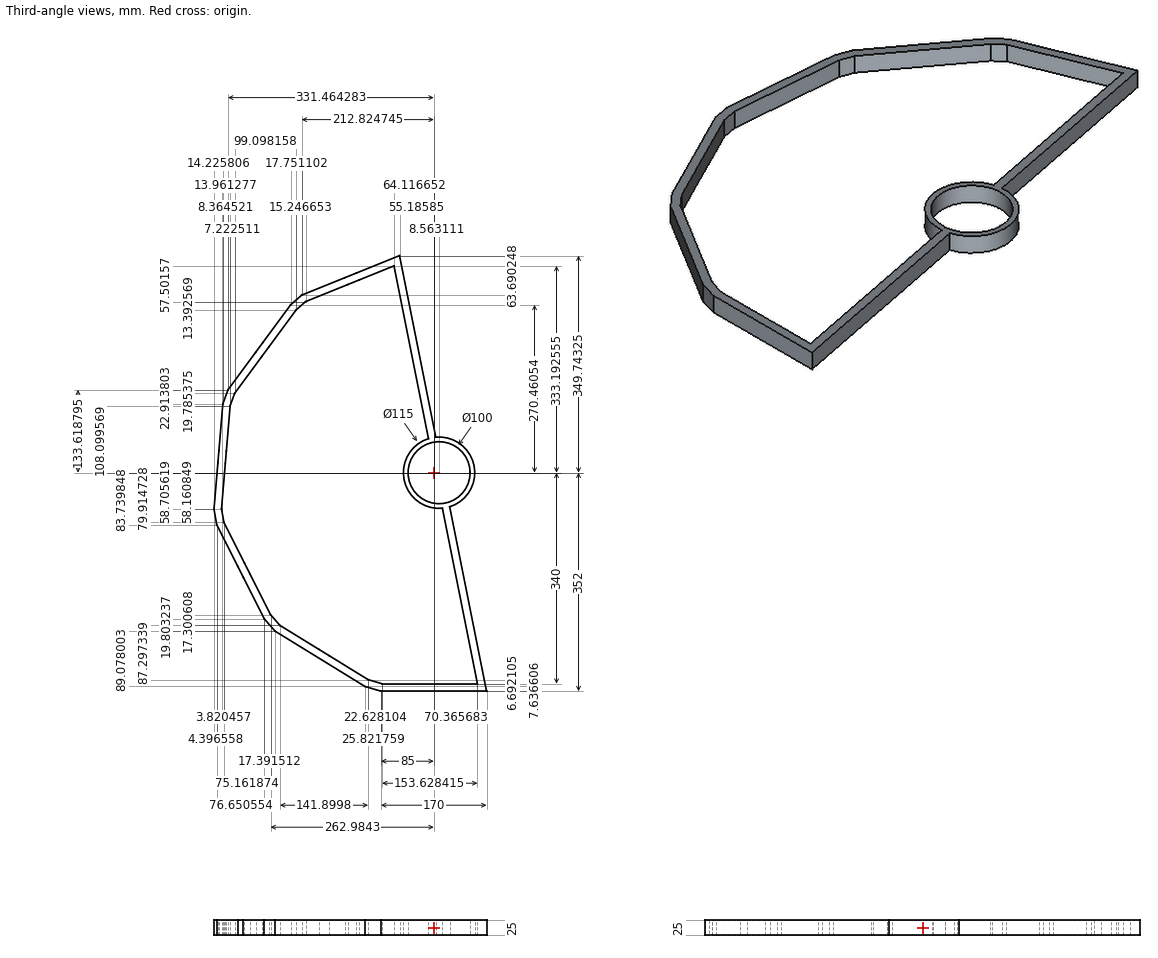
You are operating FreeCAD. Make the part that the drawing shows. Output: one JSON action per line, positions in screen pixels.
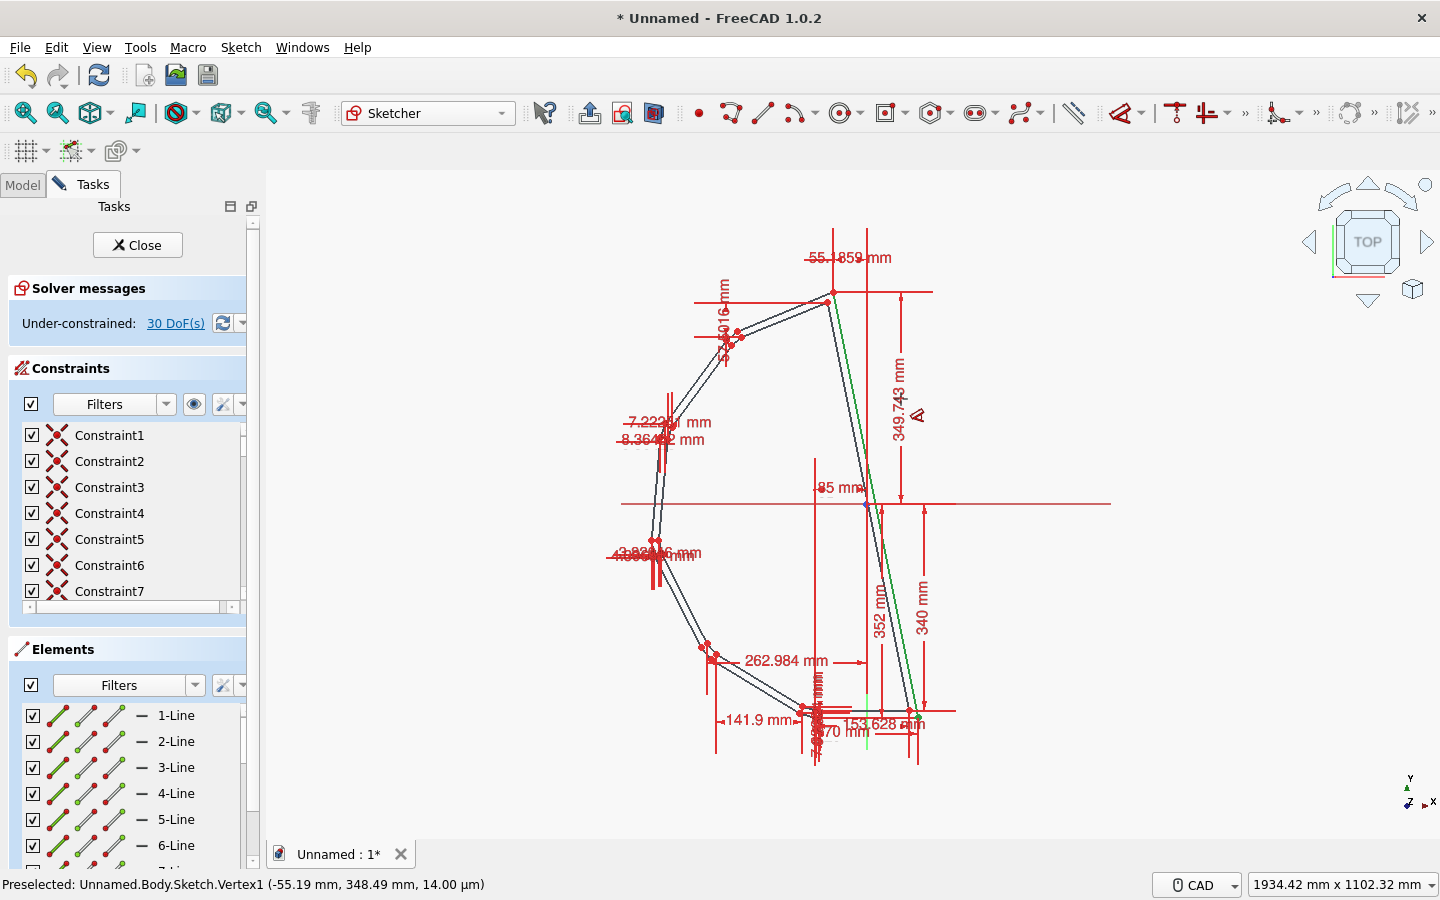
{"action": "scroll", "coordinate": [726, 341], "scroll_direction": "up", "scroll_amount": 3}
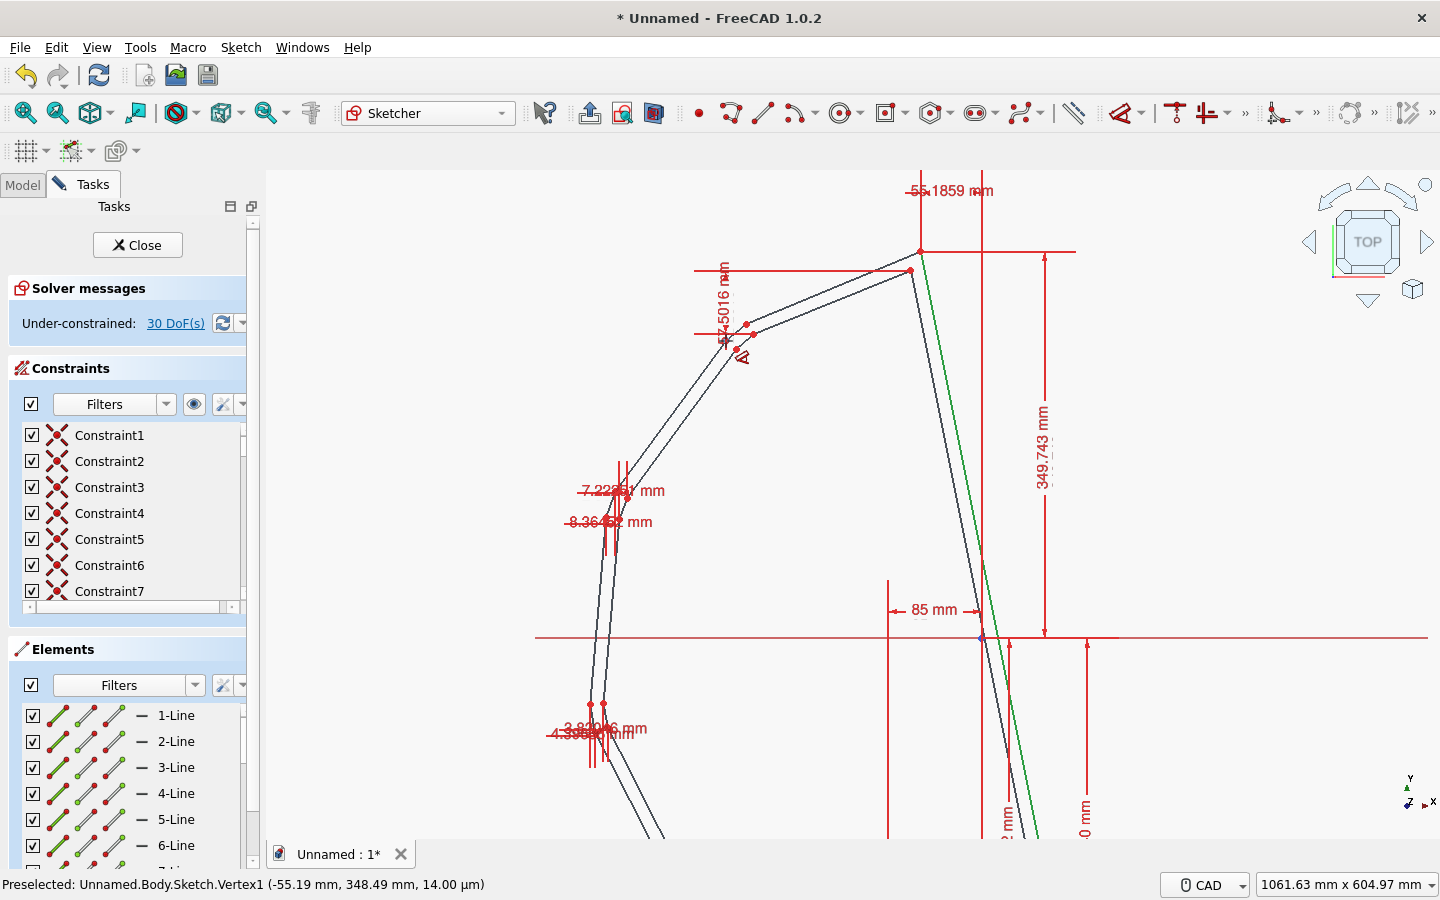
{"action": "left_click", "coordinate": [726, 340]}
{"action": "left_click", "coordinate": [1016, 489]}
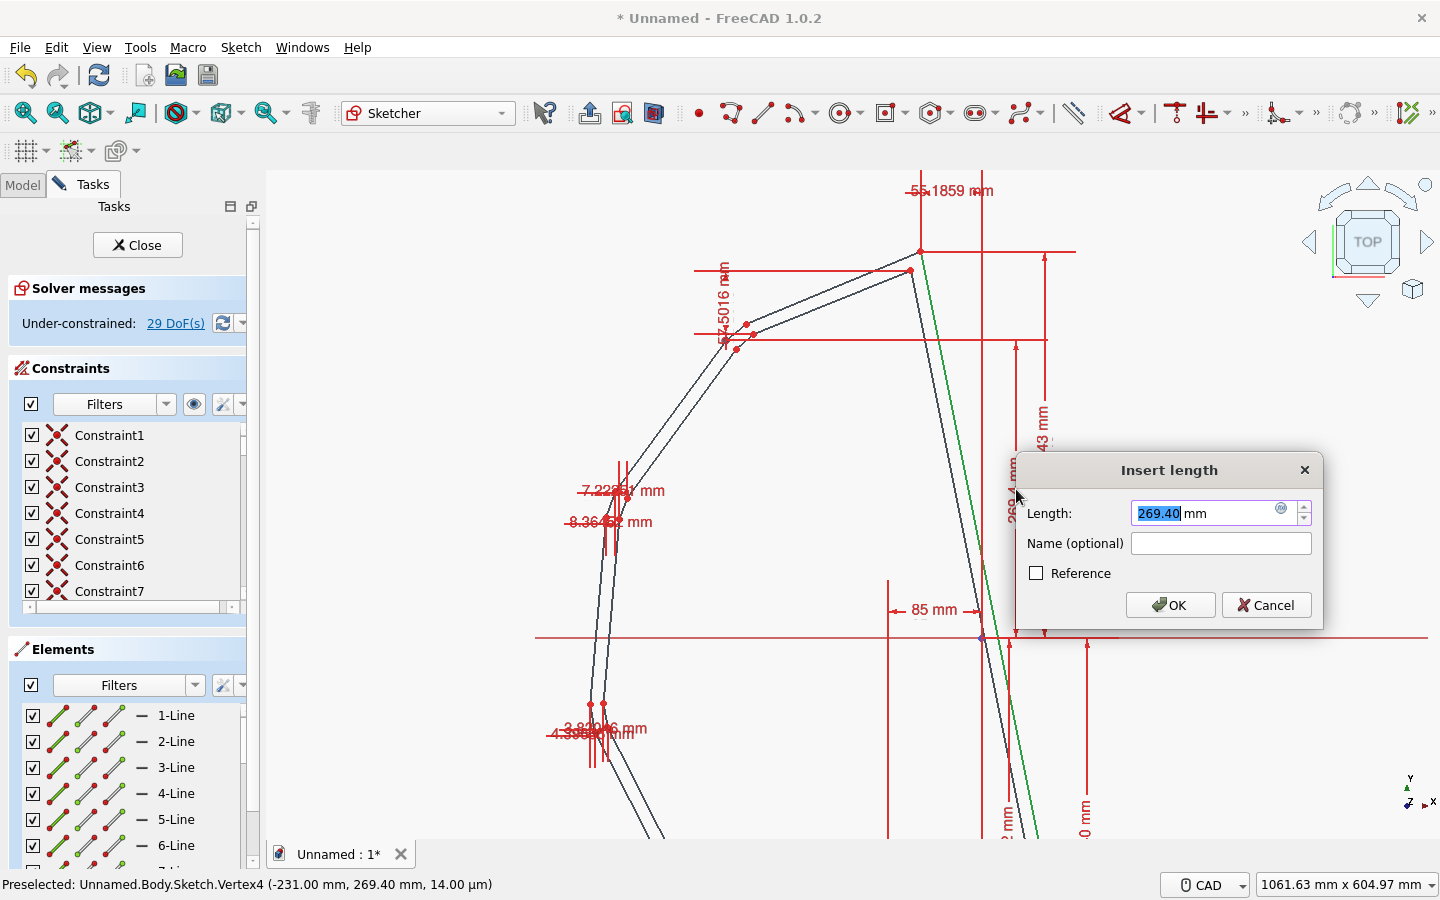
{"action": "type", "text": "270.46054"}
{"action": "key", "text": "Return"}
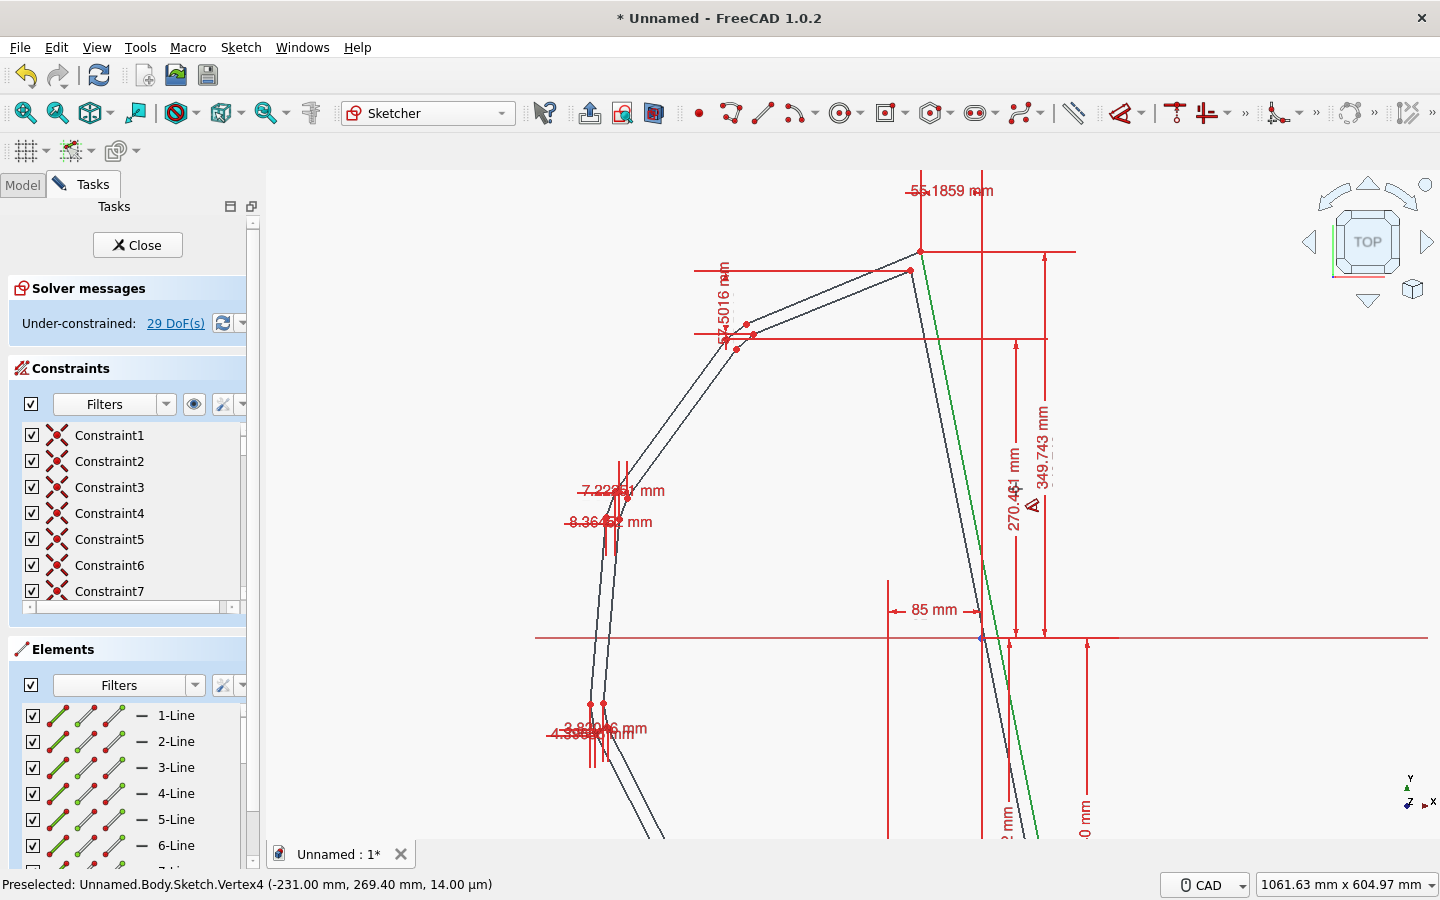
{"action": "left_click", "coordinate": [590, 705]}
{"action": "left_click", "coordinate": [556, 672]}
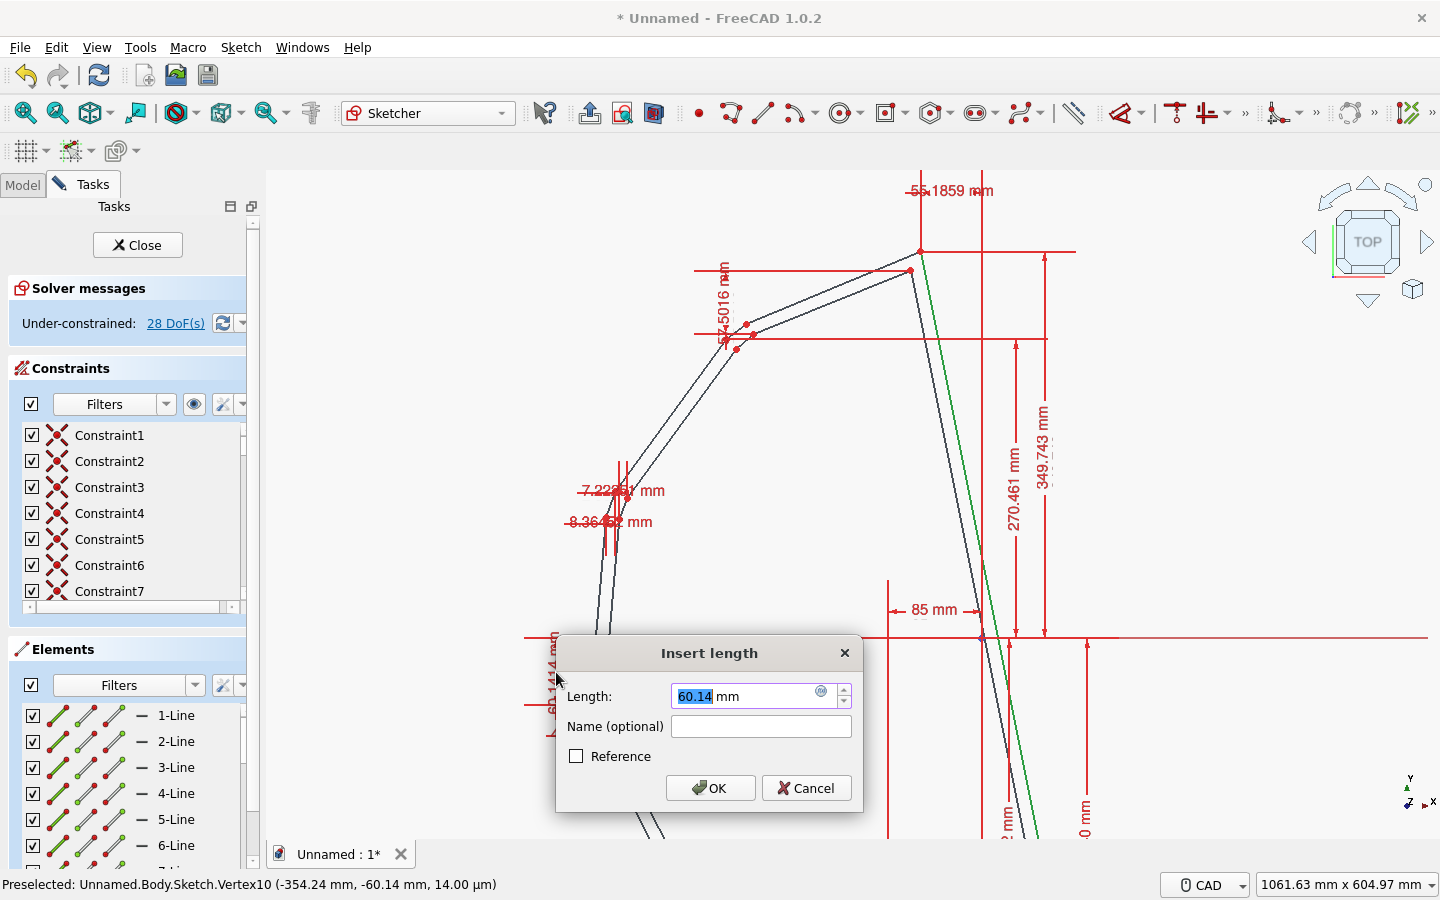
{"action": "type", "text": "58.705619"}
{"action": "key", "text": "Return"}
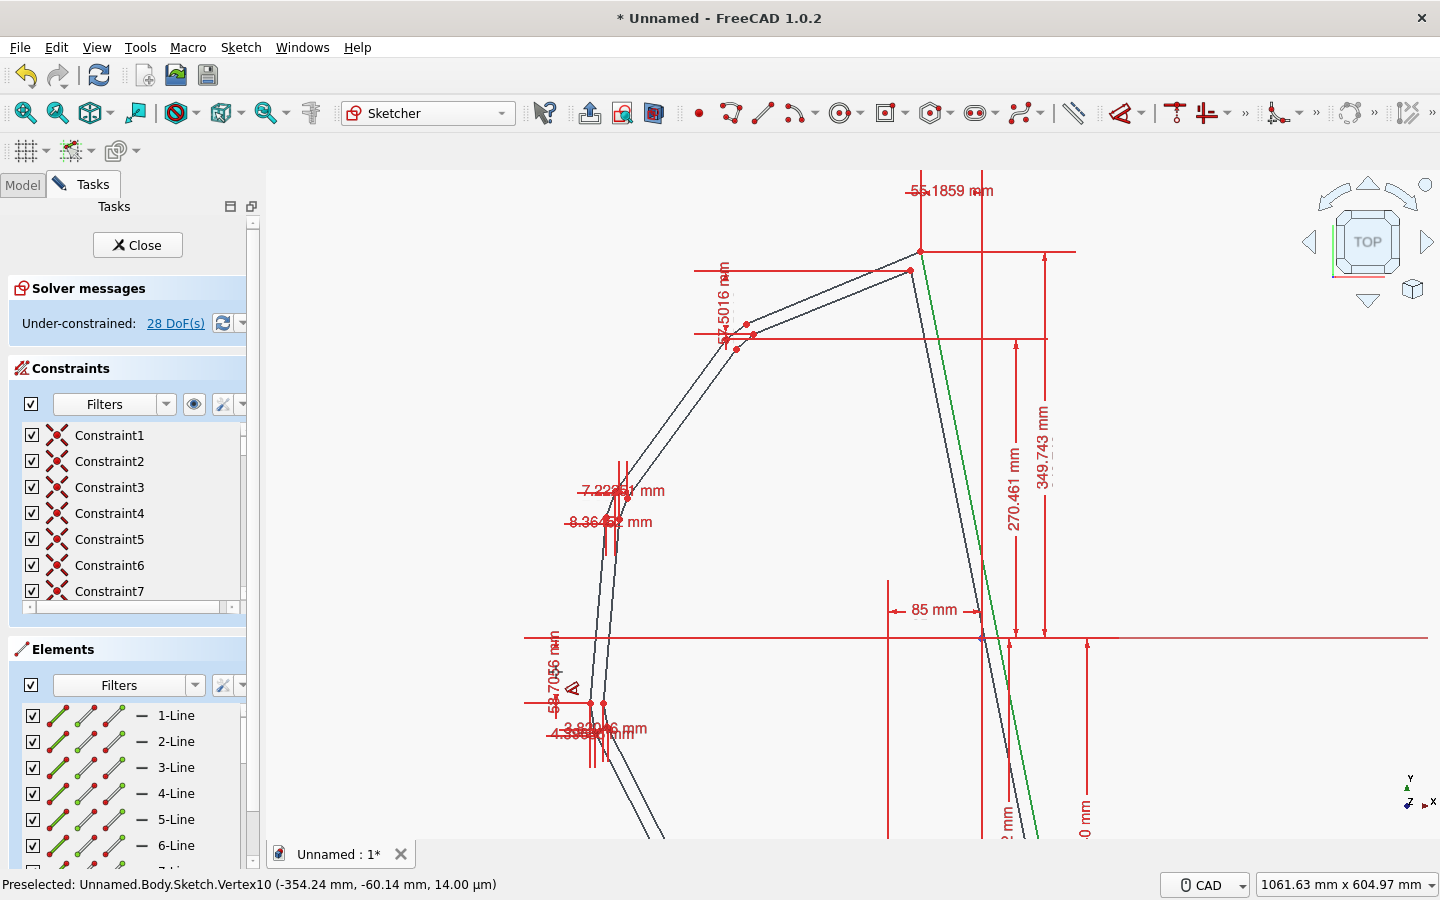
{"action": "left_click", "coordinate": [595, 732]}
{"action": "left_click", "coordinate": [561, 707]}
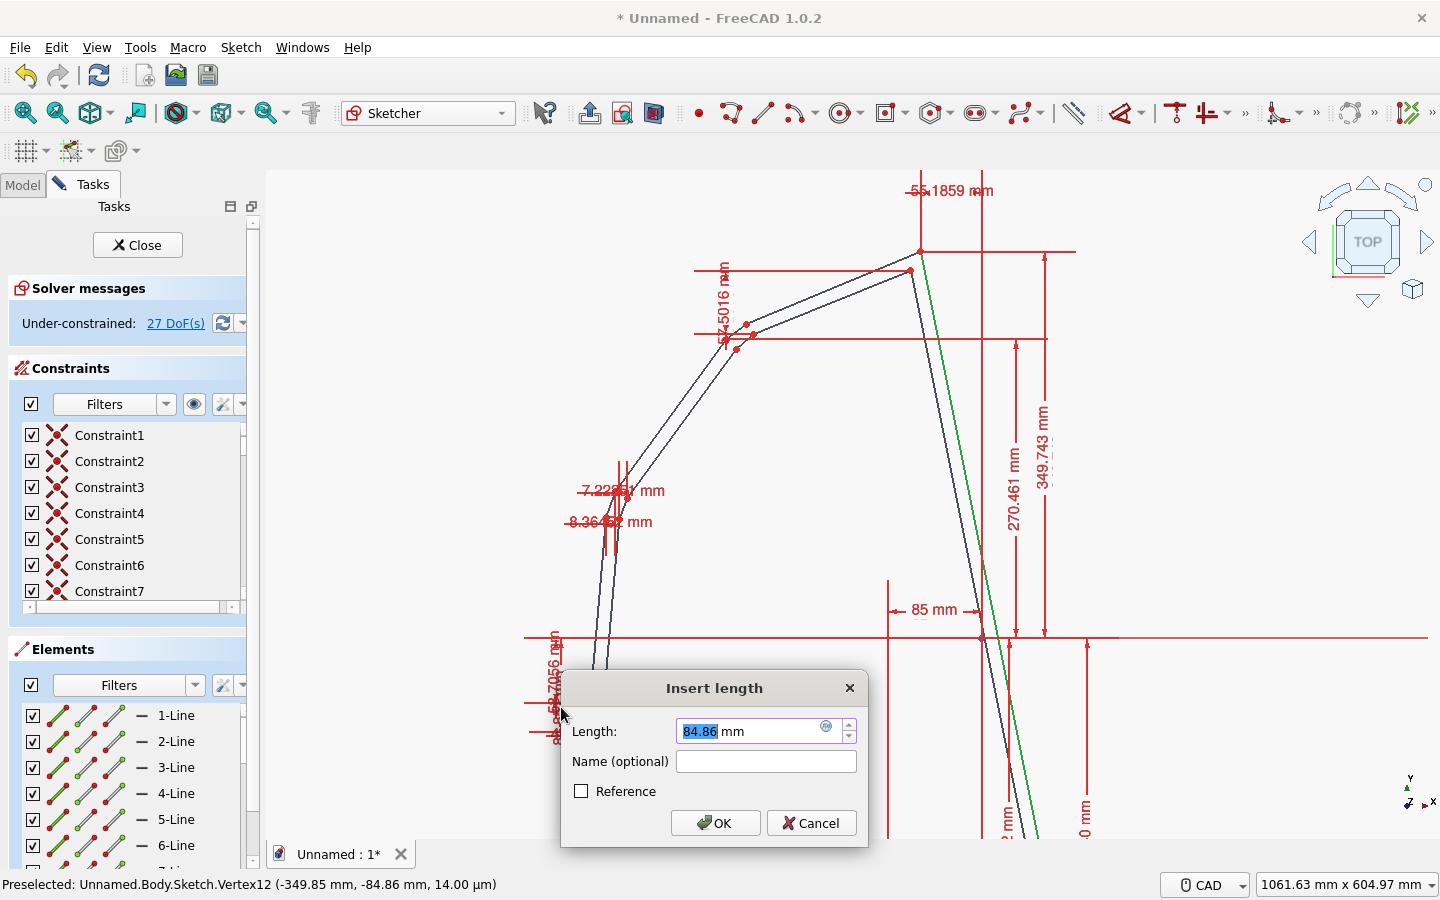
{"action": "type", "text": "83.739848"}
{"action": "key", "text": "Return"}